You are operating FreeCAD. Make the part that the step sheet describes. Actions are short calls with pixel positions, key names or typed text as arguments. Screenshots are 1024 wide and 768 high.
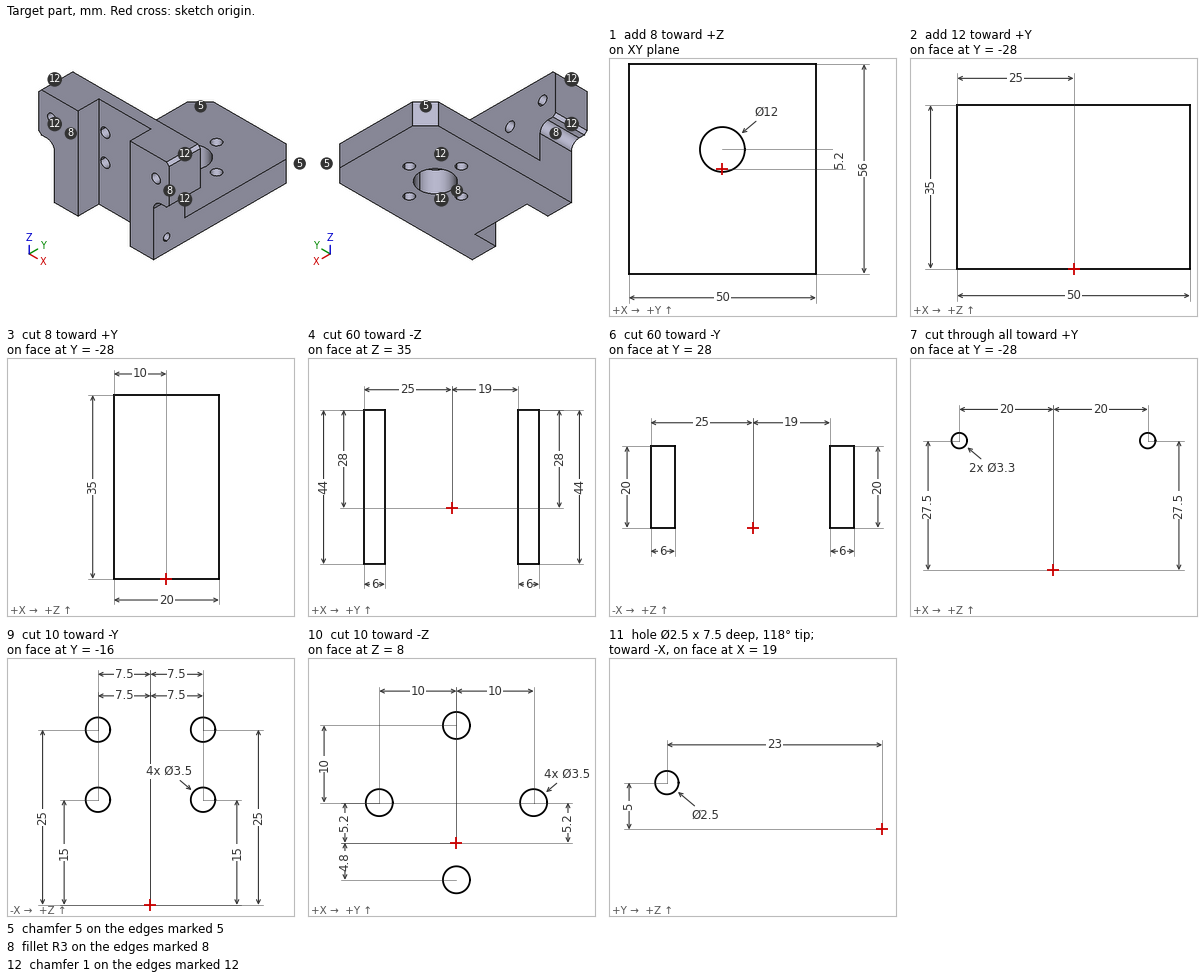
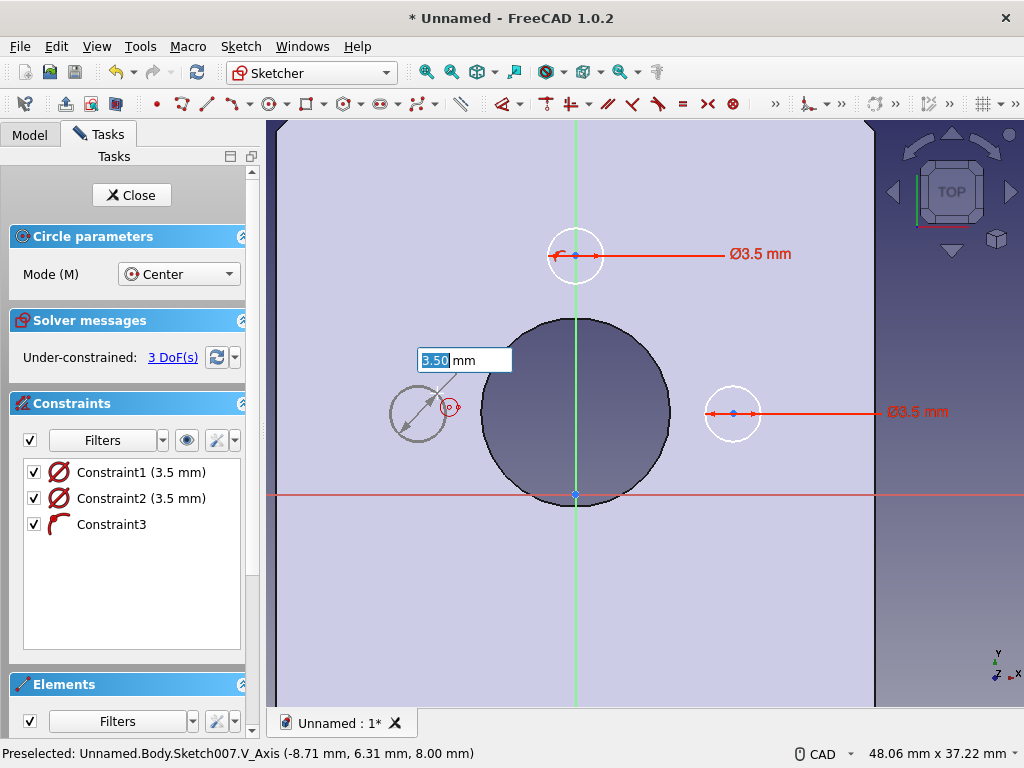
text(3.5)
key(Return)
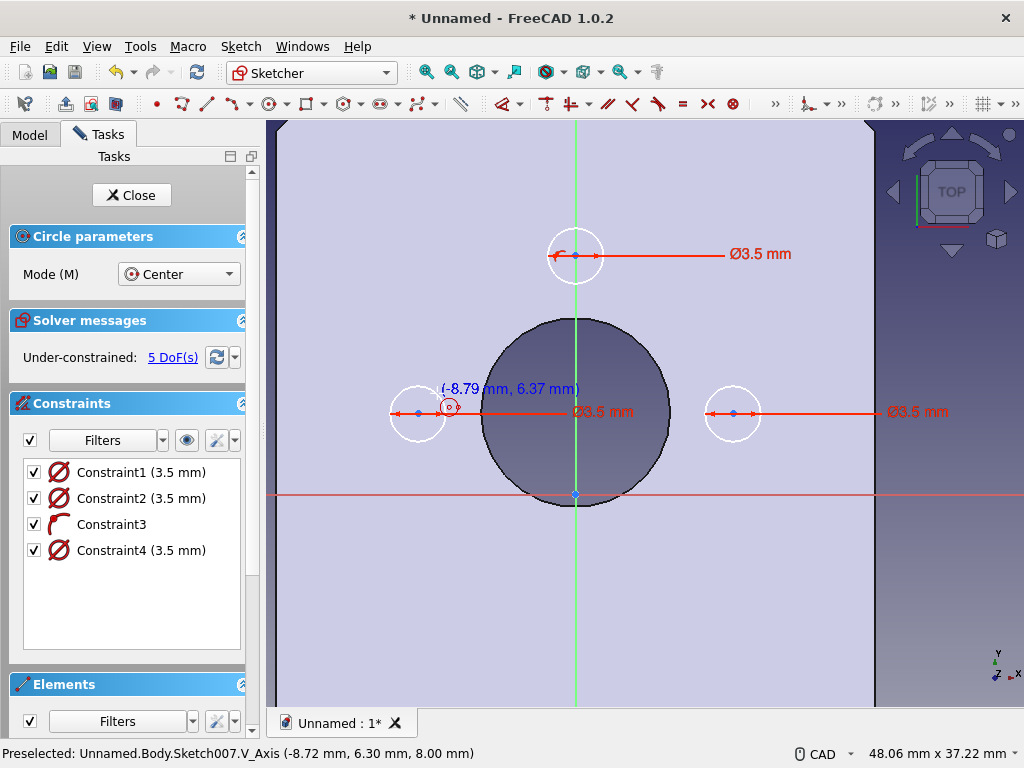
click(576, 570)
move(595, 551)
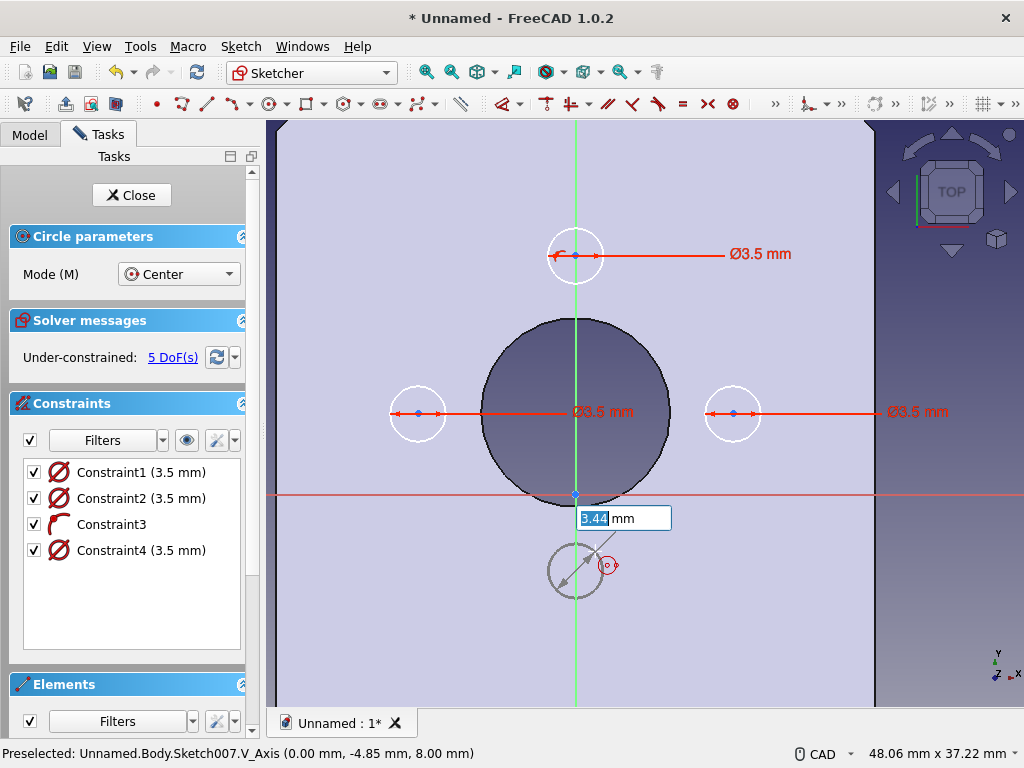
text(3.5)
key(Return)
key(Escape)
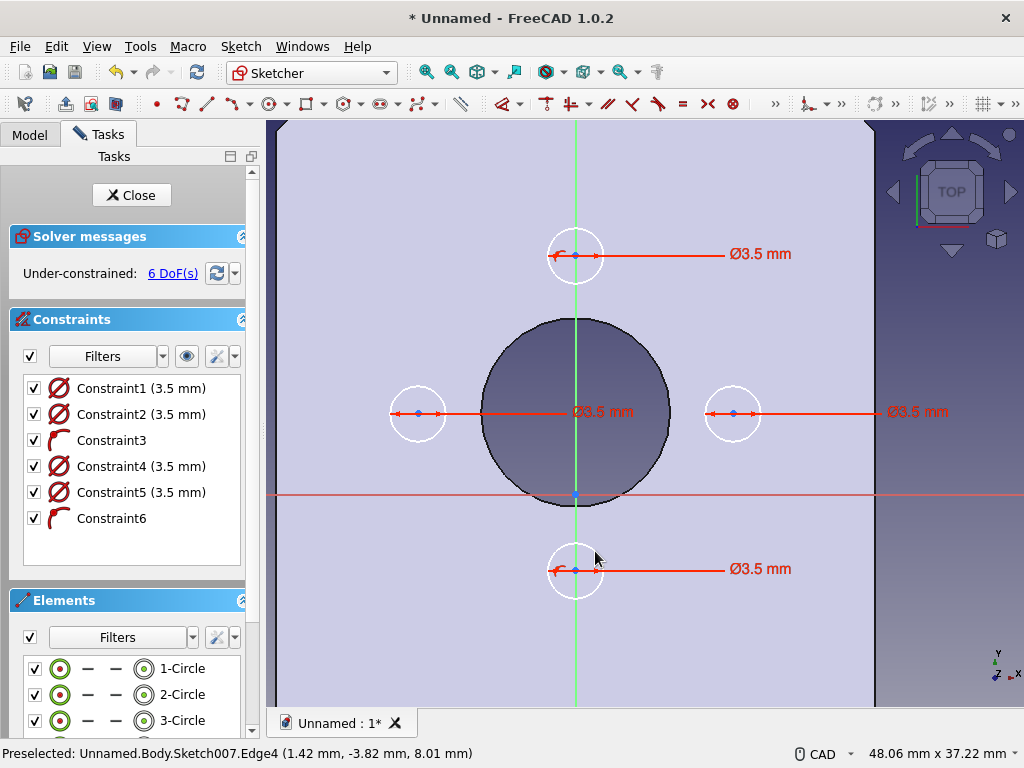
click(502, 104)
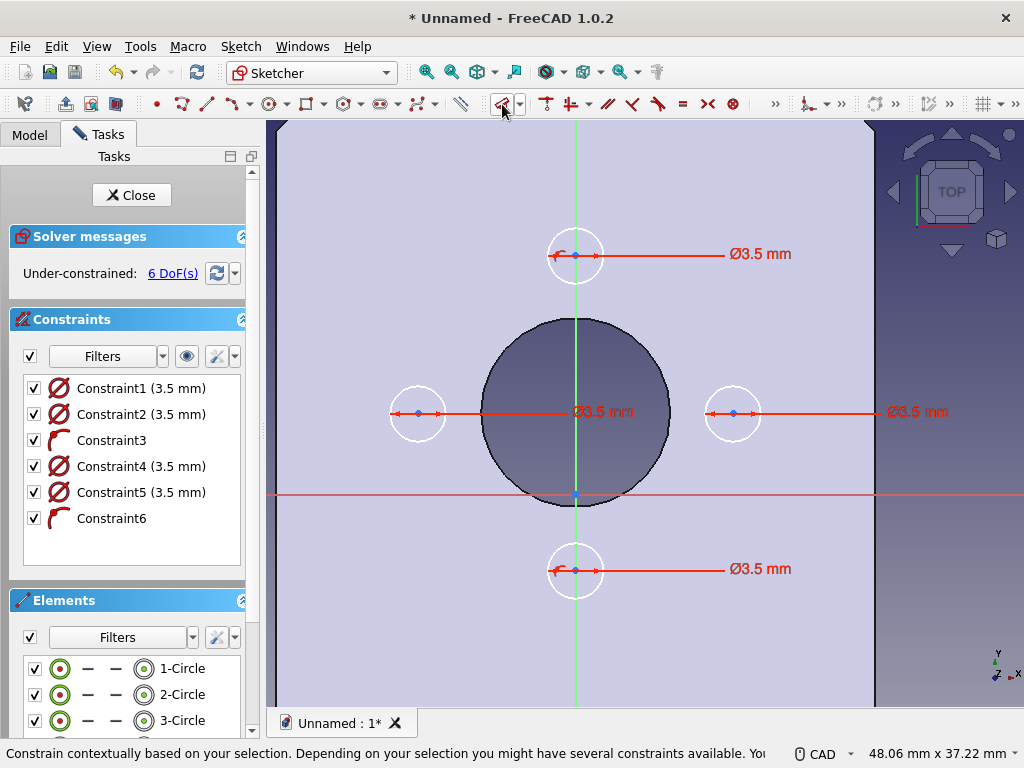
click(733, 414)
click(654, 529)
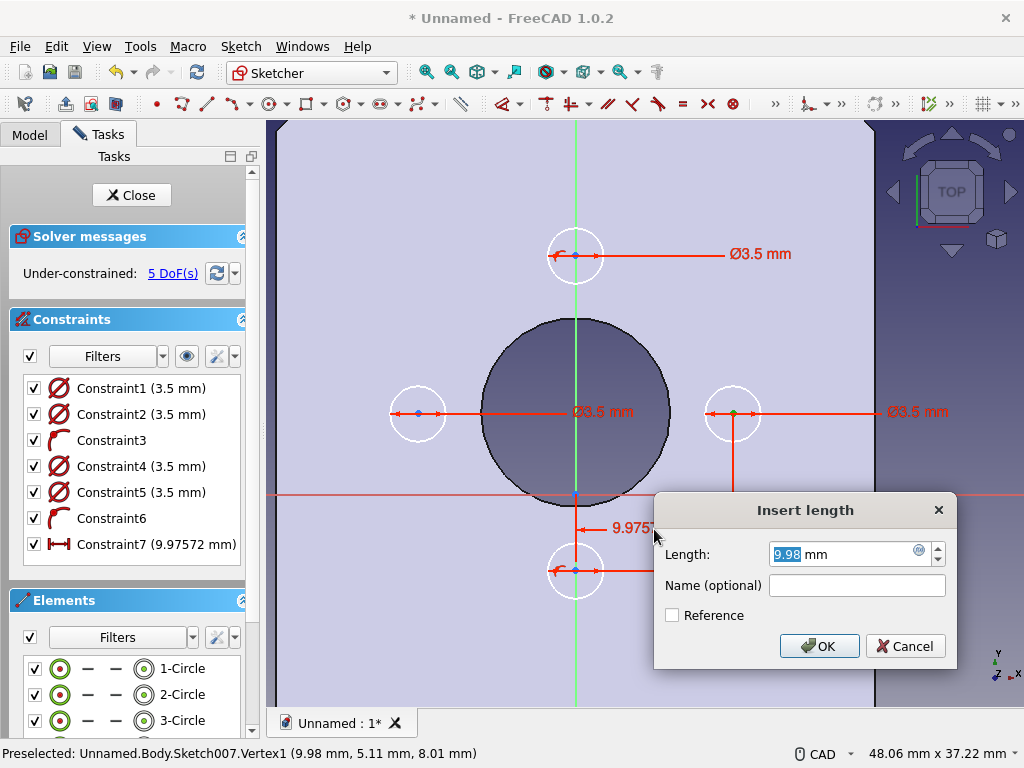
text(10)
key(Return)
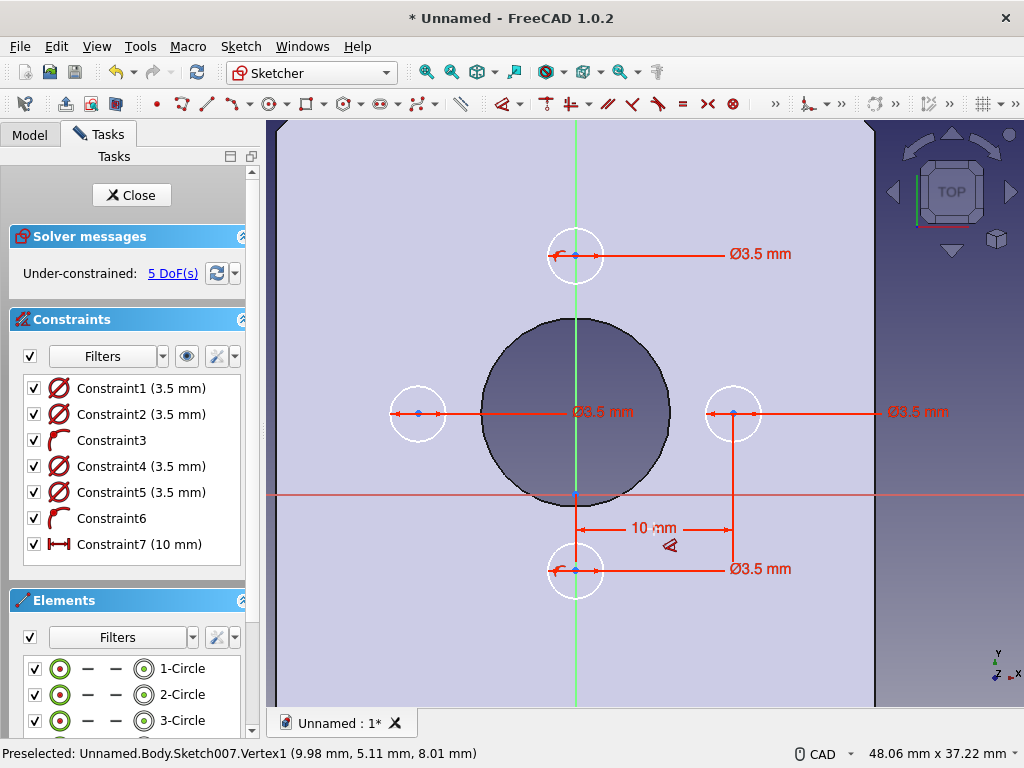
click(418, 414)
click(497, 529)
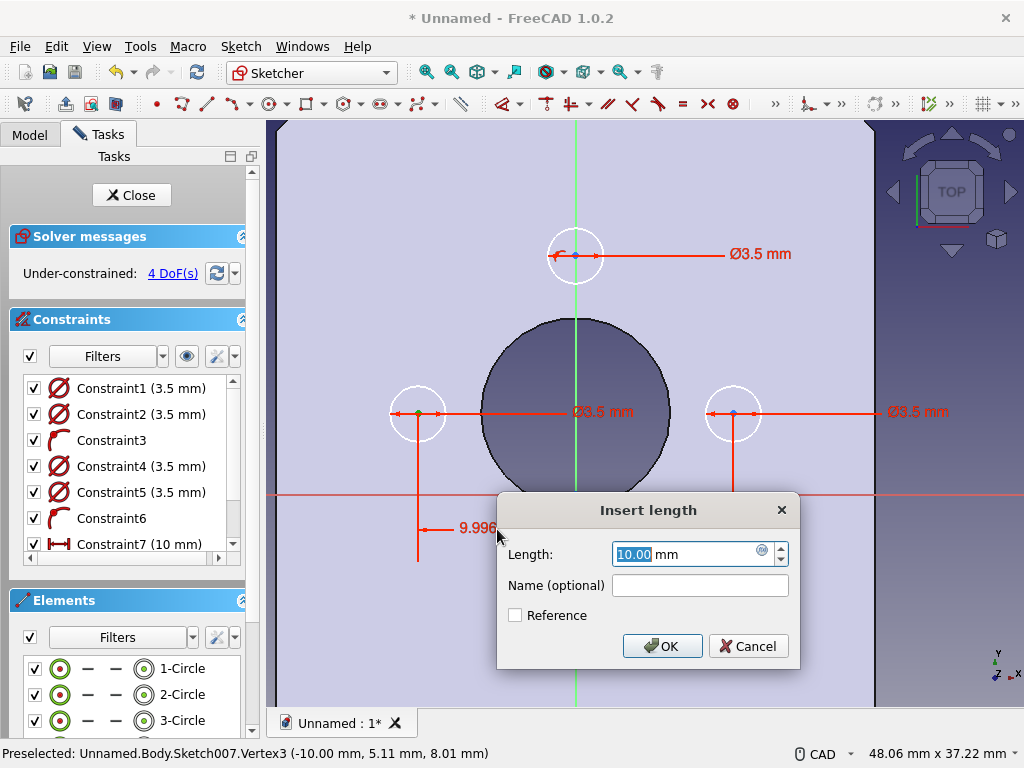
text(10)
key(Return)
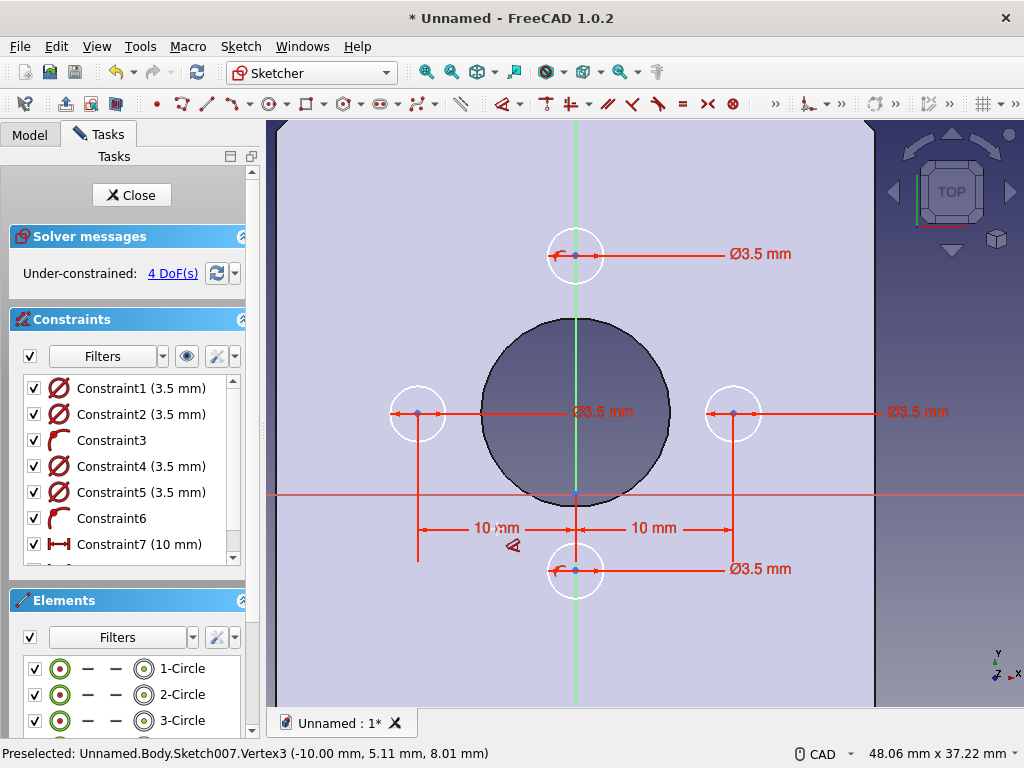
click(733, 414)
click(767, 454)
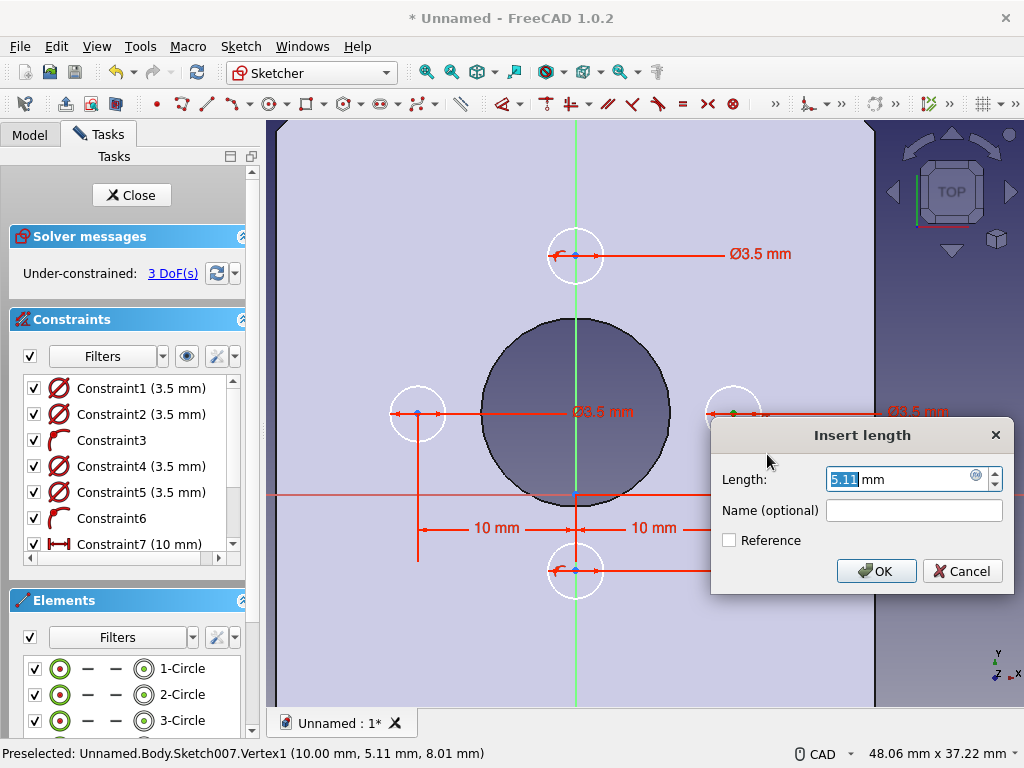
text(5.2)
key(Return)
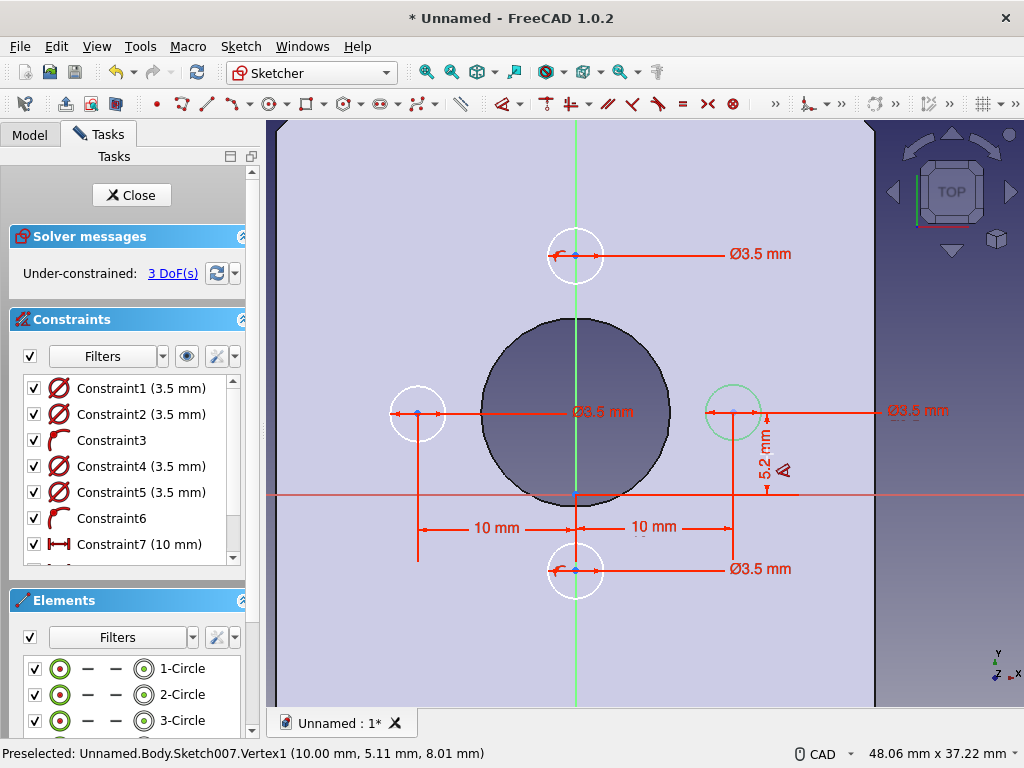
click(418, 414)
click(384, 454)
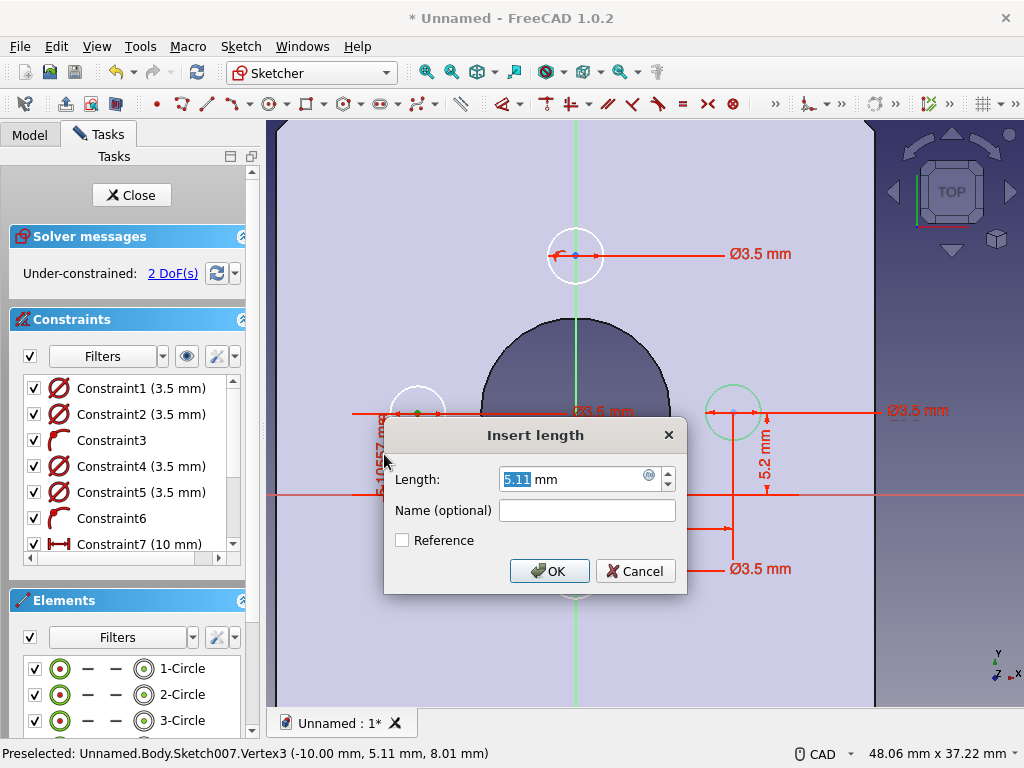
text(5.2)
key(Return)